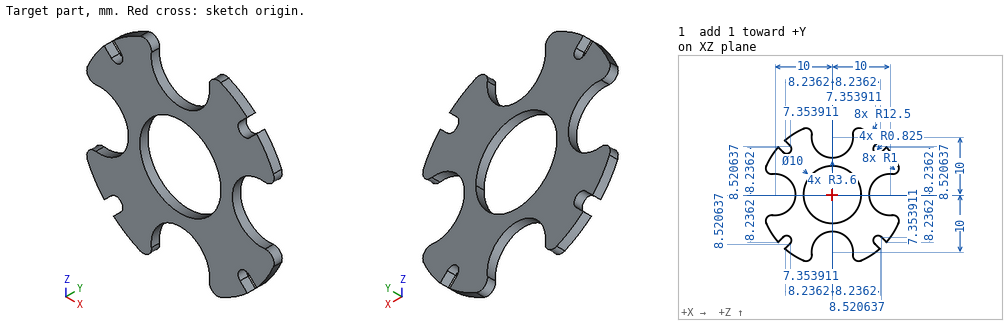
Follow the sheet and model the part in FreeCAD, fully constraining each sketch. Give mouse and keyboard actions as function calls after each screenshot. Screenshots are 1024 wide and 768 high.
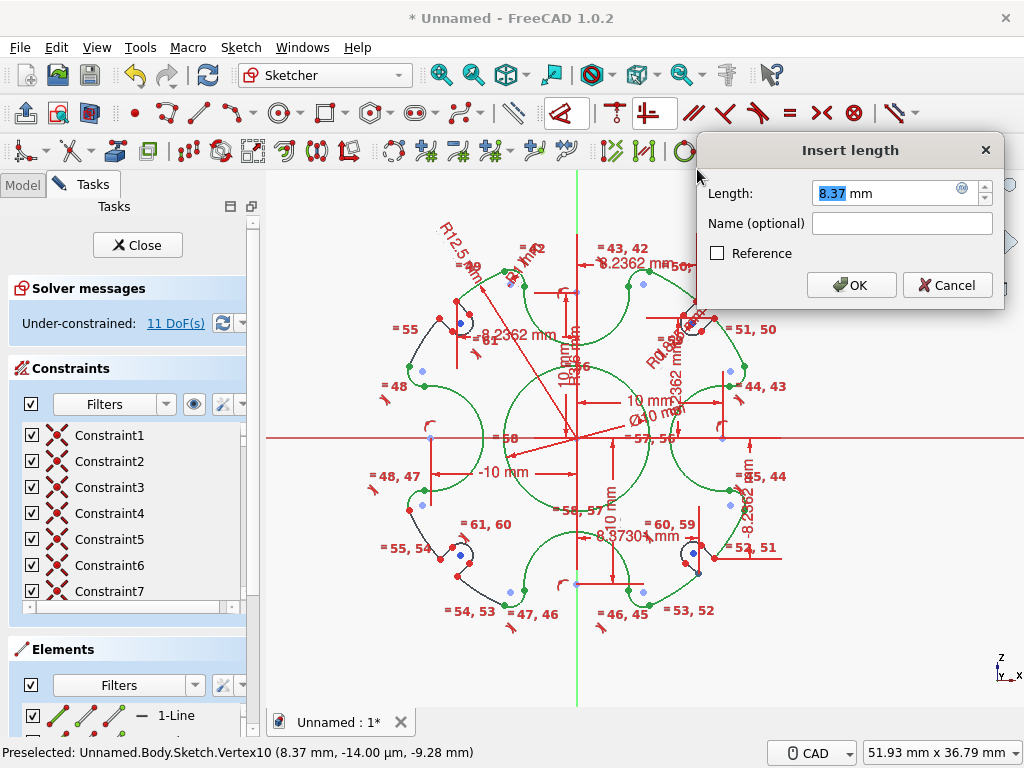
text(8.2362)
key(Return)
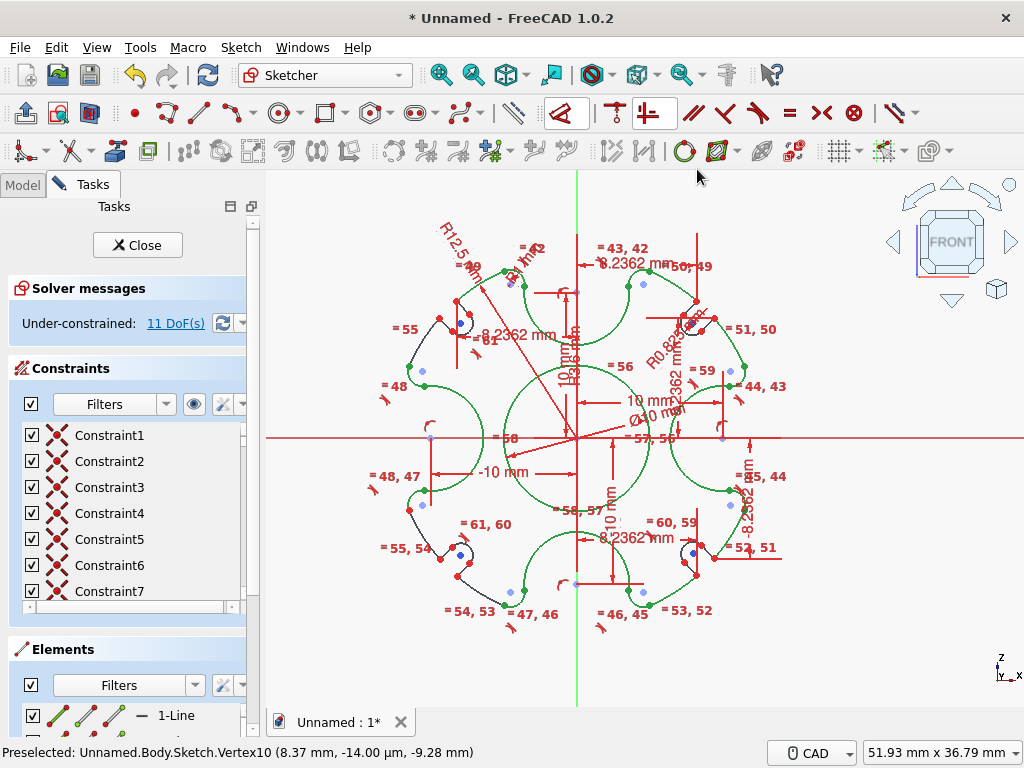
click(457, 576)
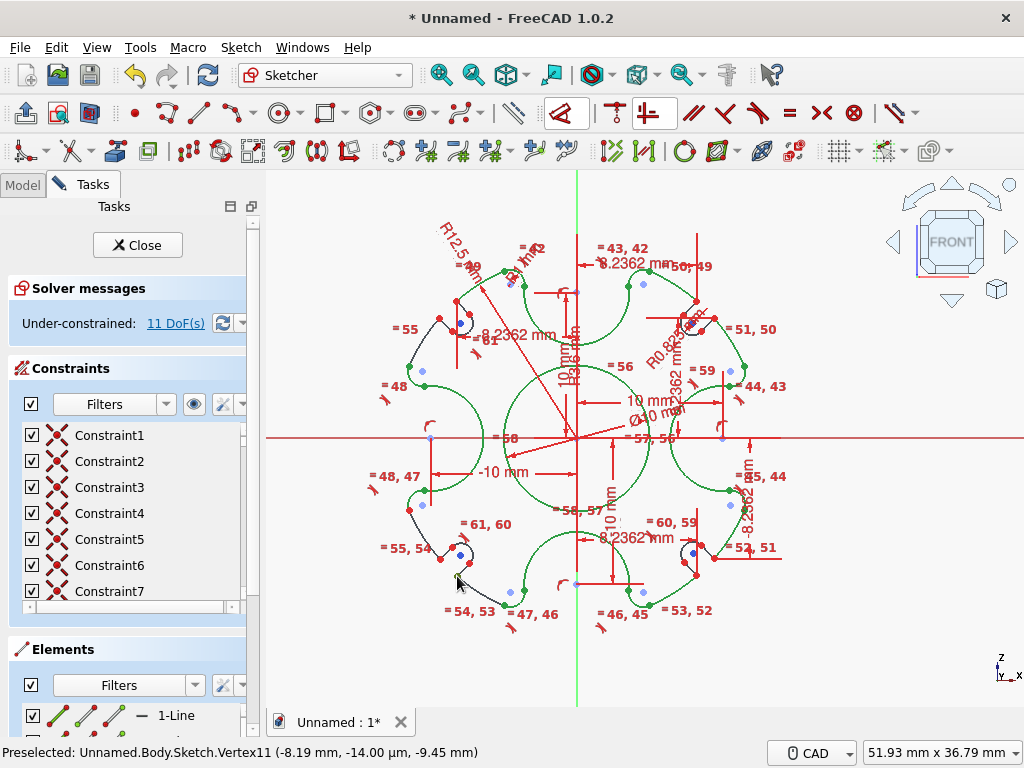
key(l)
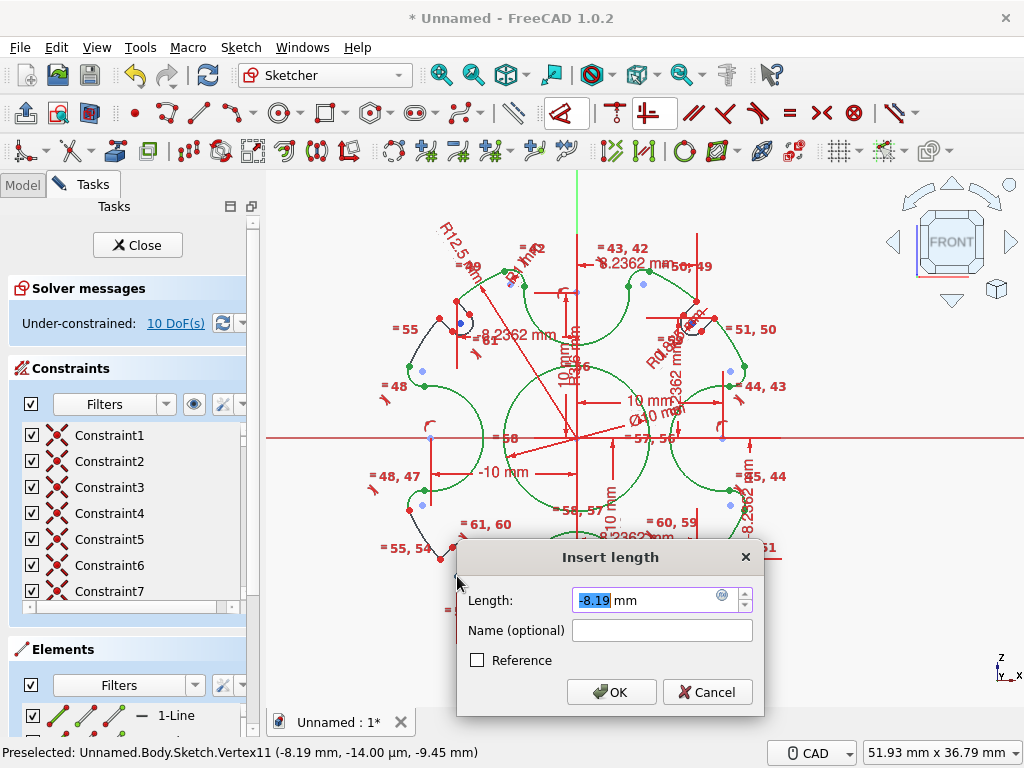
text(-8.2362)
key(Return)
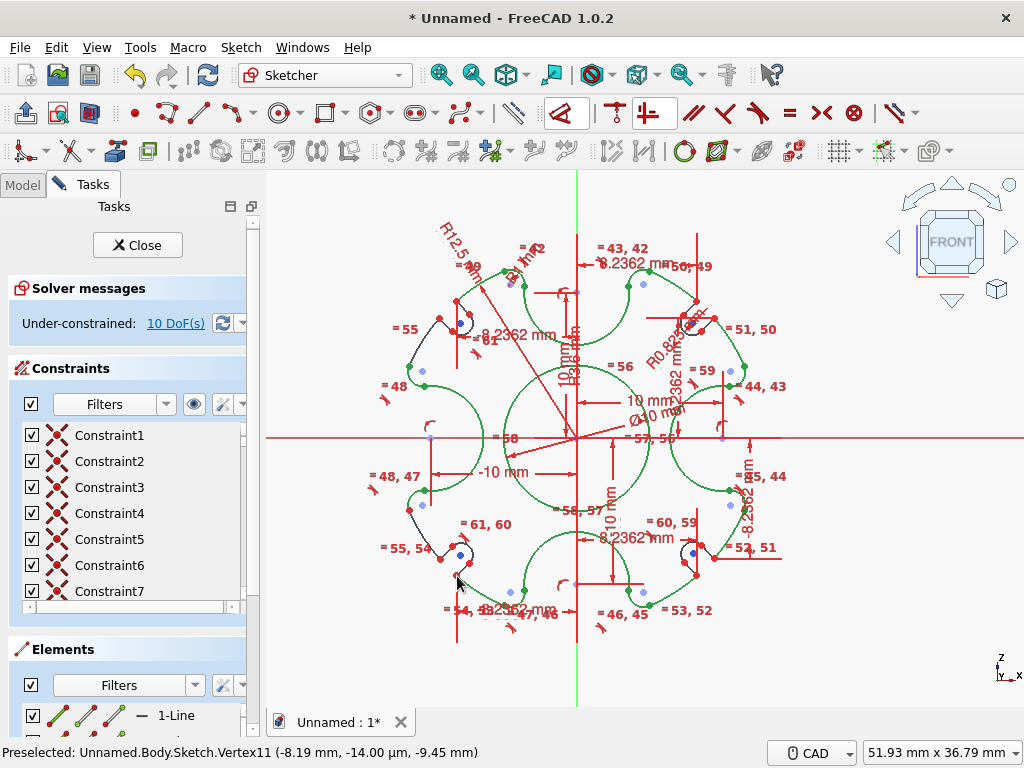
click(440, 560)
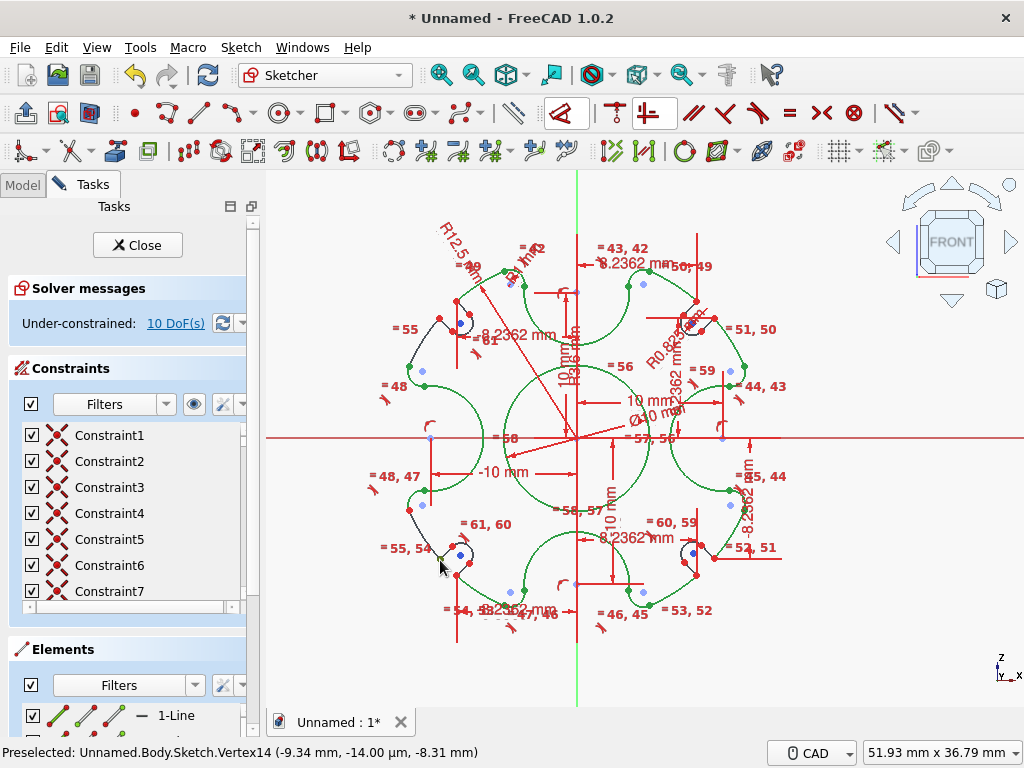
key(i)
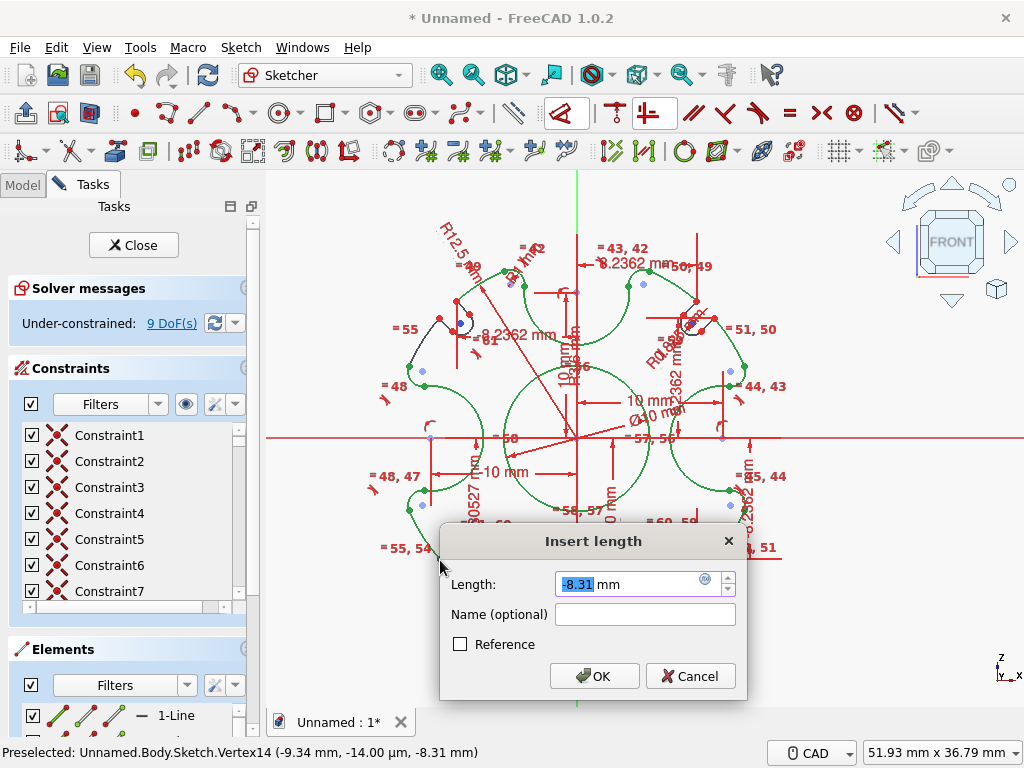
text(-8.2362)
key(Return)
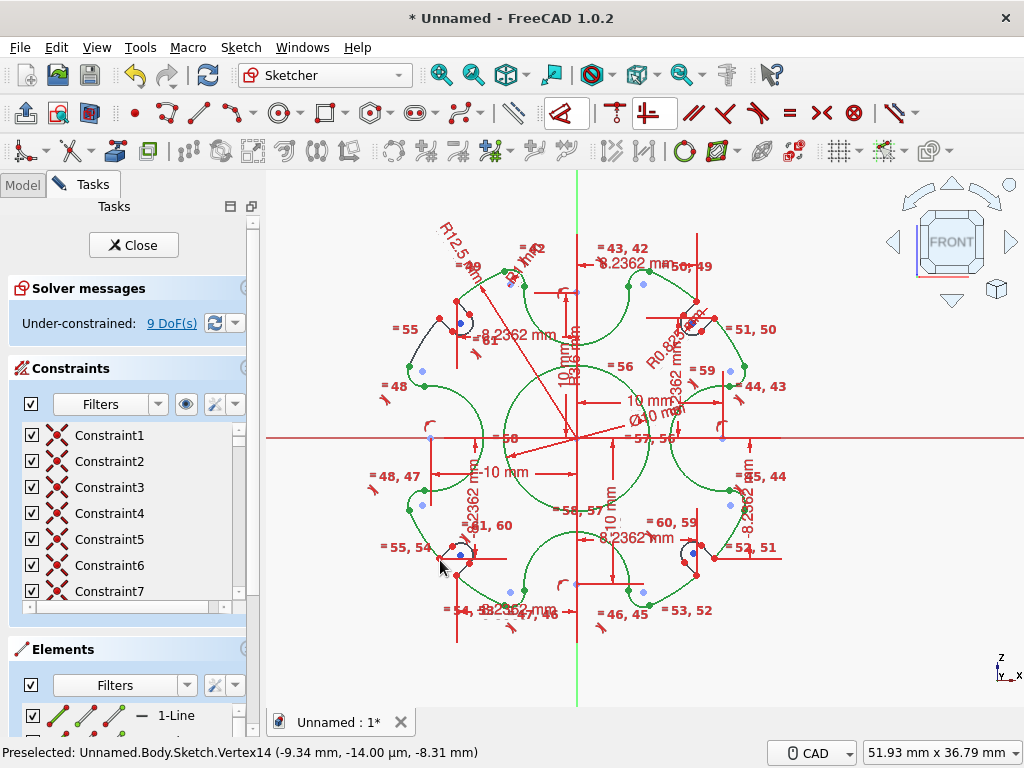
click(439, 319)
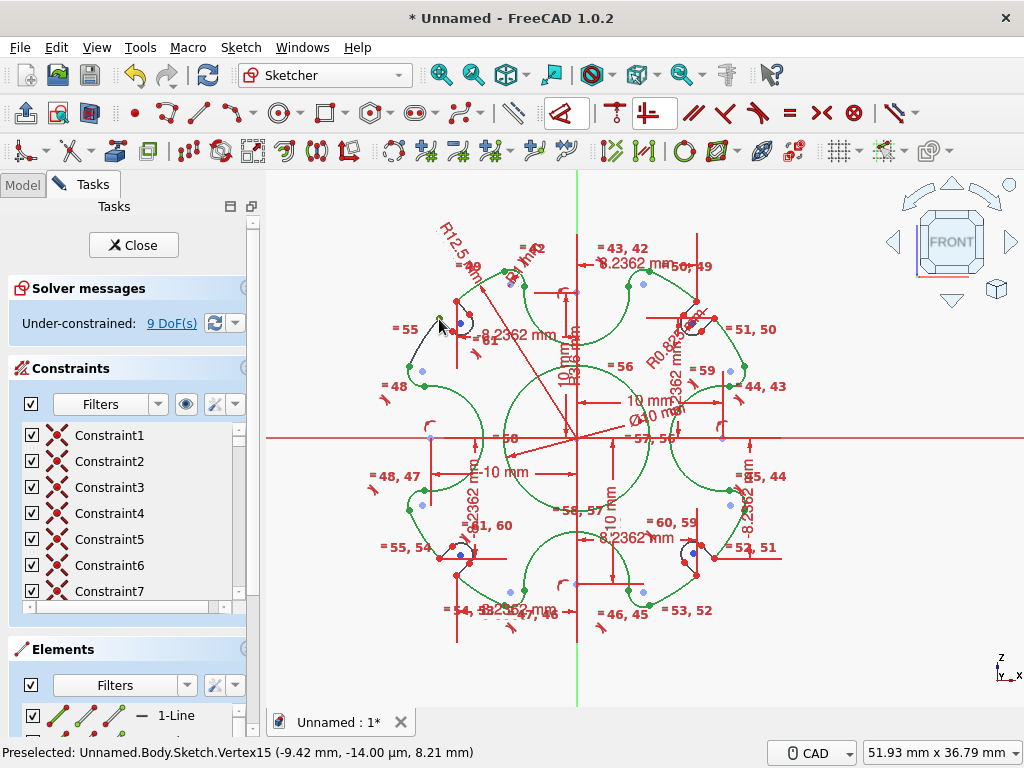
click(584, 114)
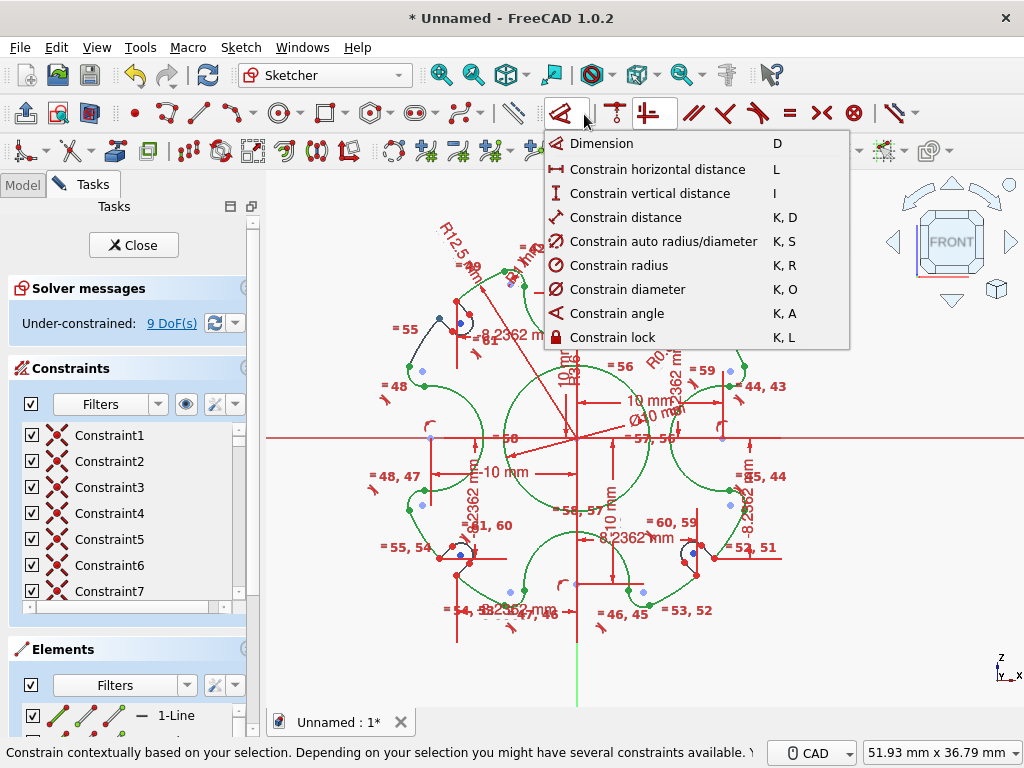
click(697, 193)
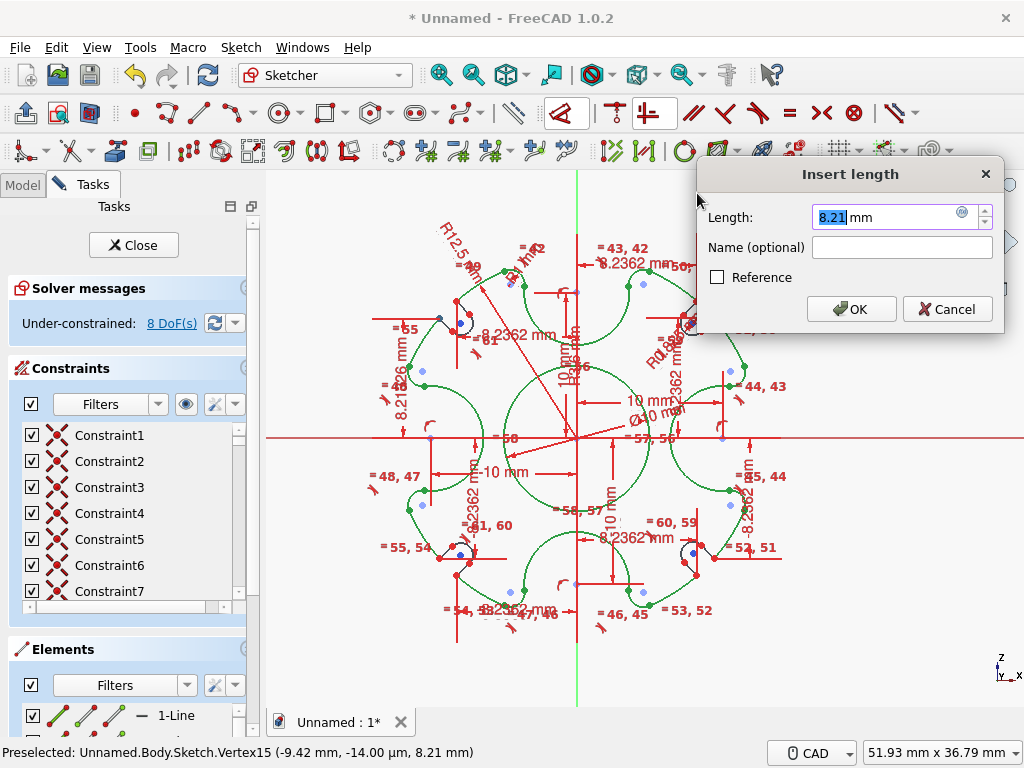
text(8.2362)
key(Return)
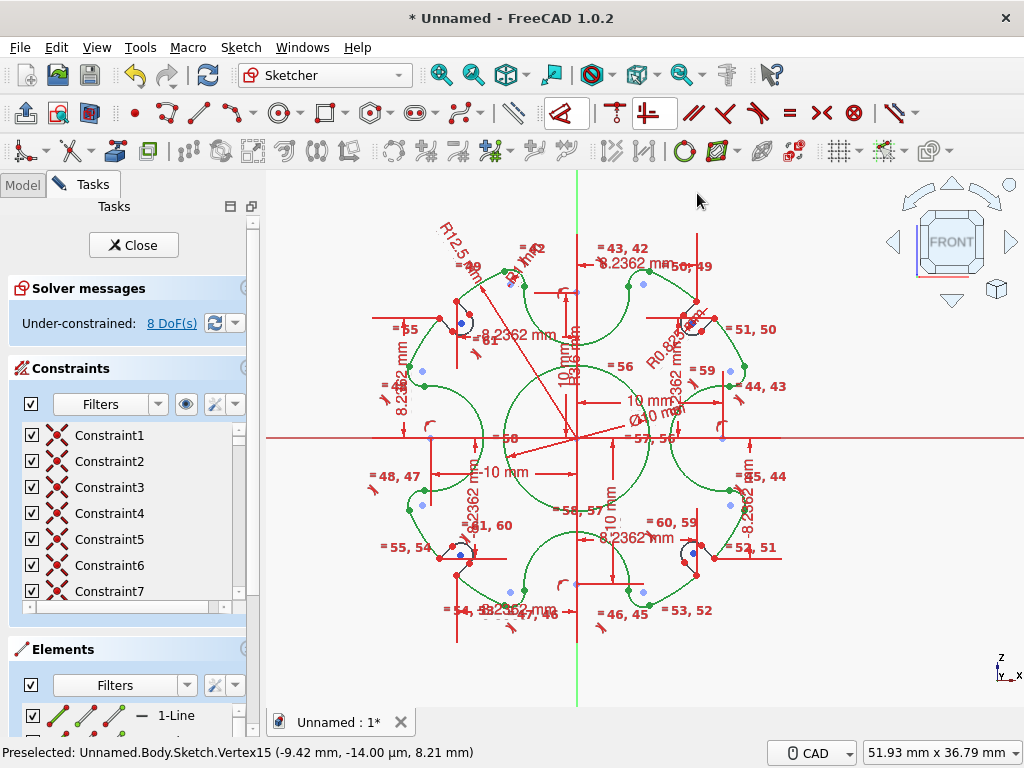
click(470, 315)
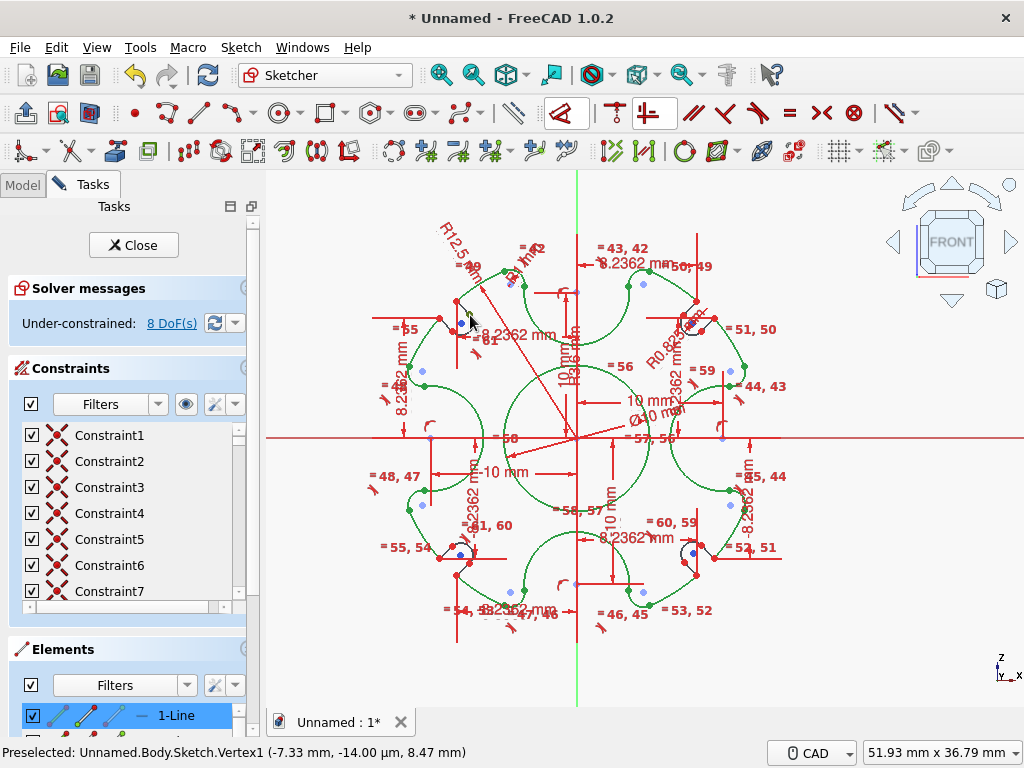
click(584, 114)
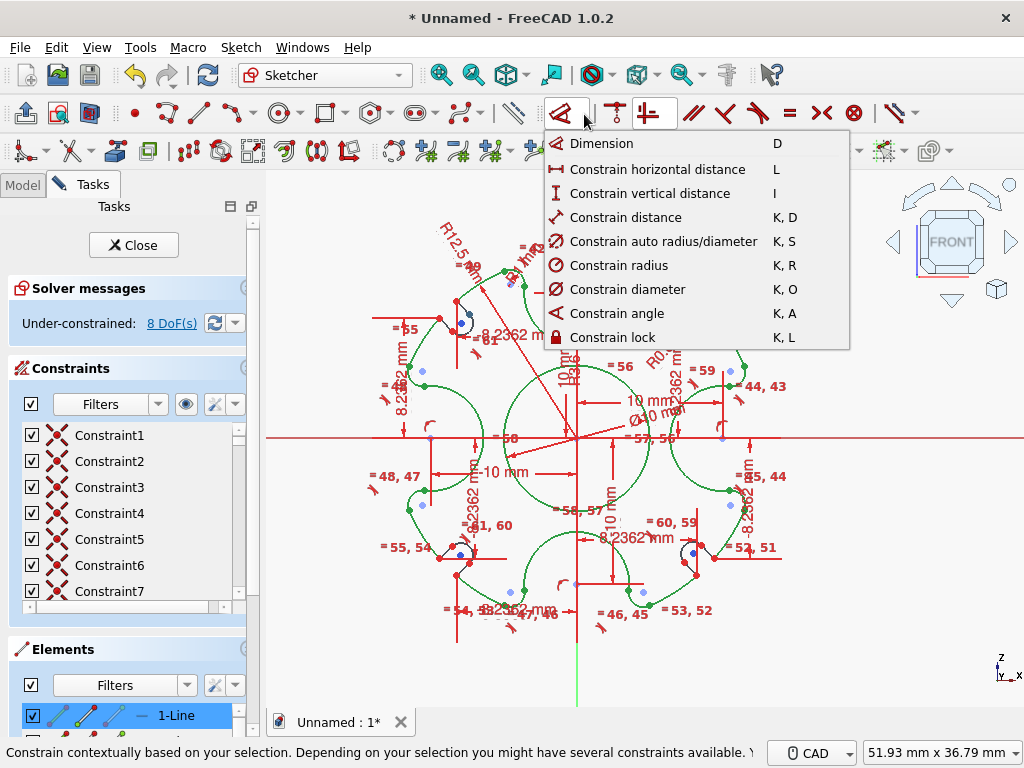
click(697, 169)